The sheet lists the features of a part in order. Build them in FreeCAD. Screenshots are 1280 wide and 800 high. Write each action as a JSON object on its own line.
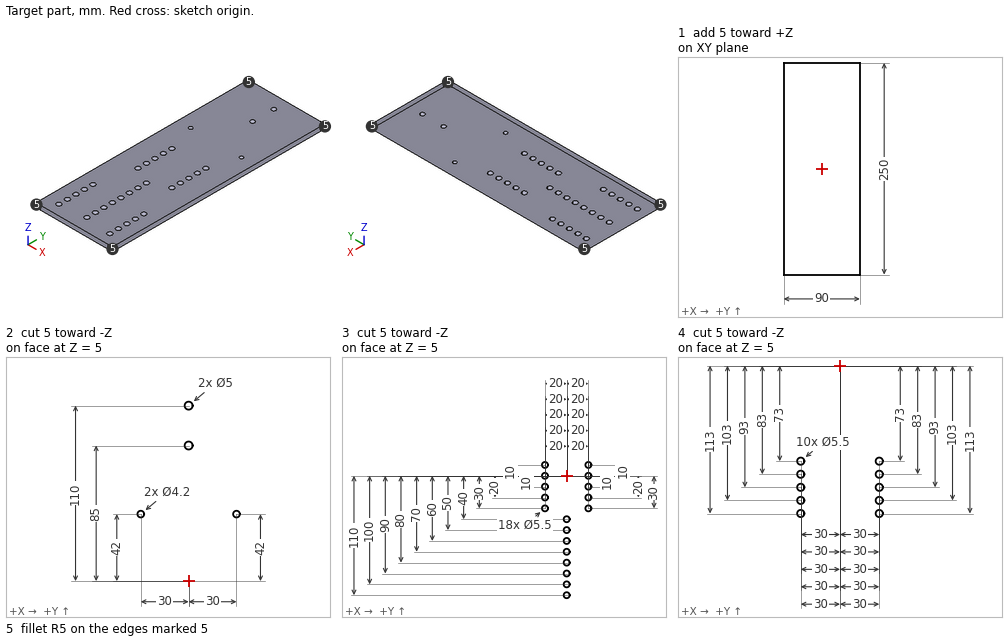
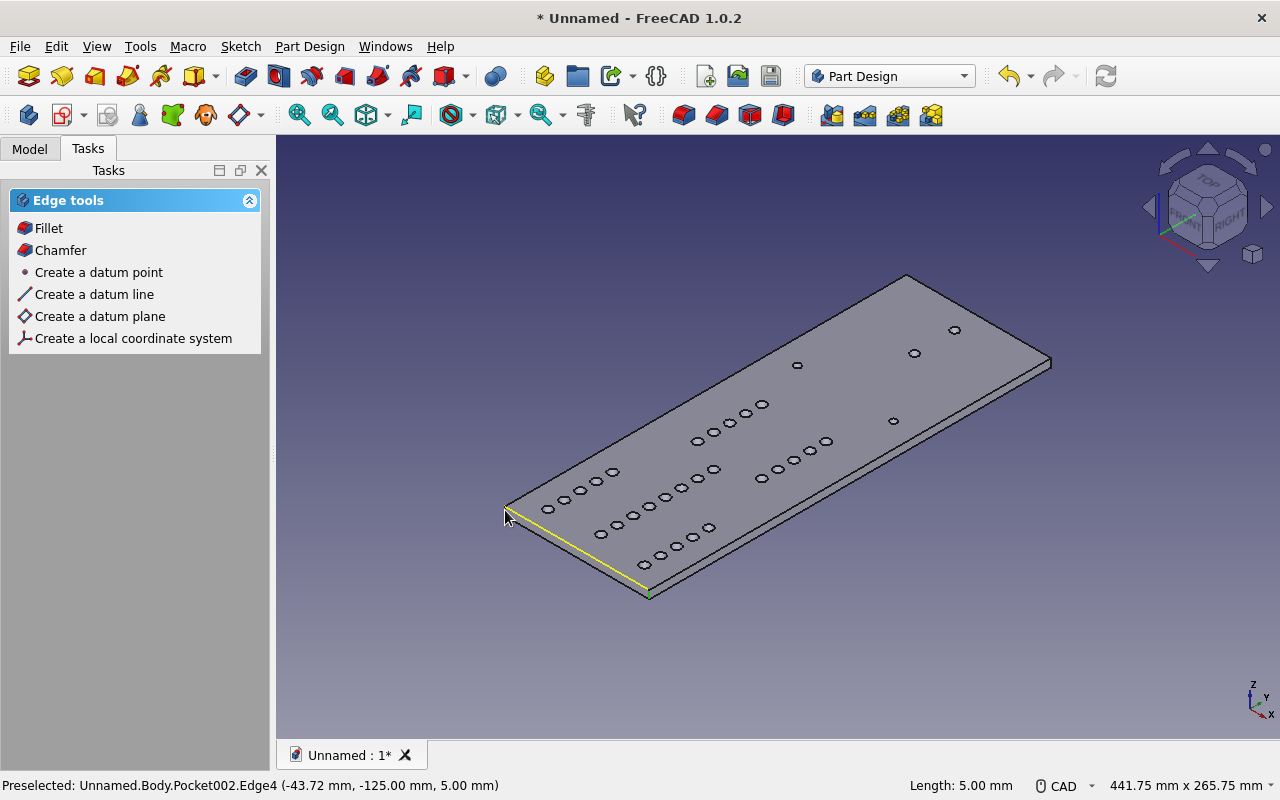
{"action": "key", "text": "2"}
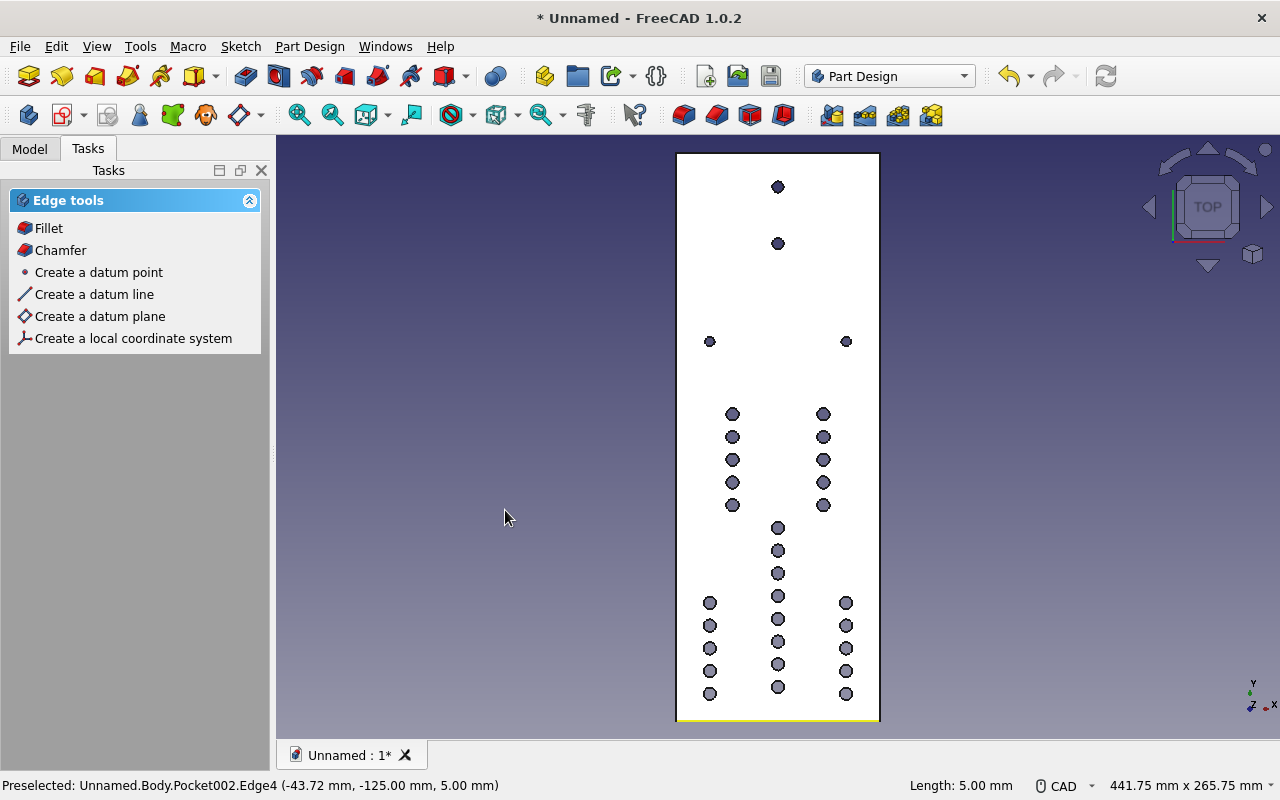
{"action": "key", "text": "1"}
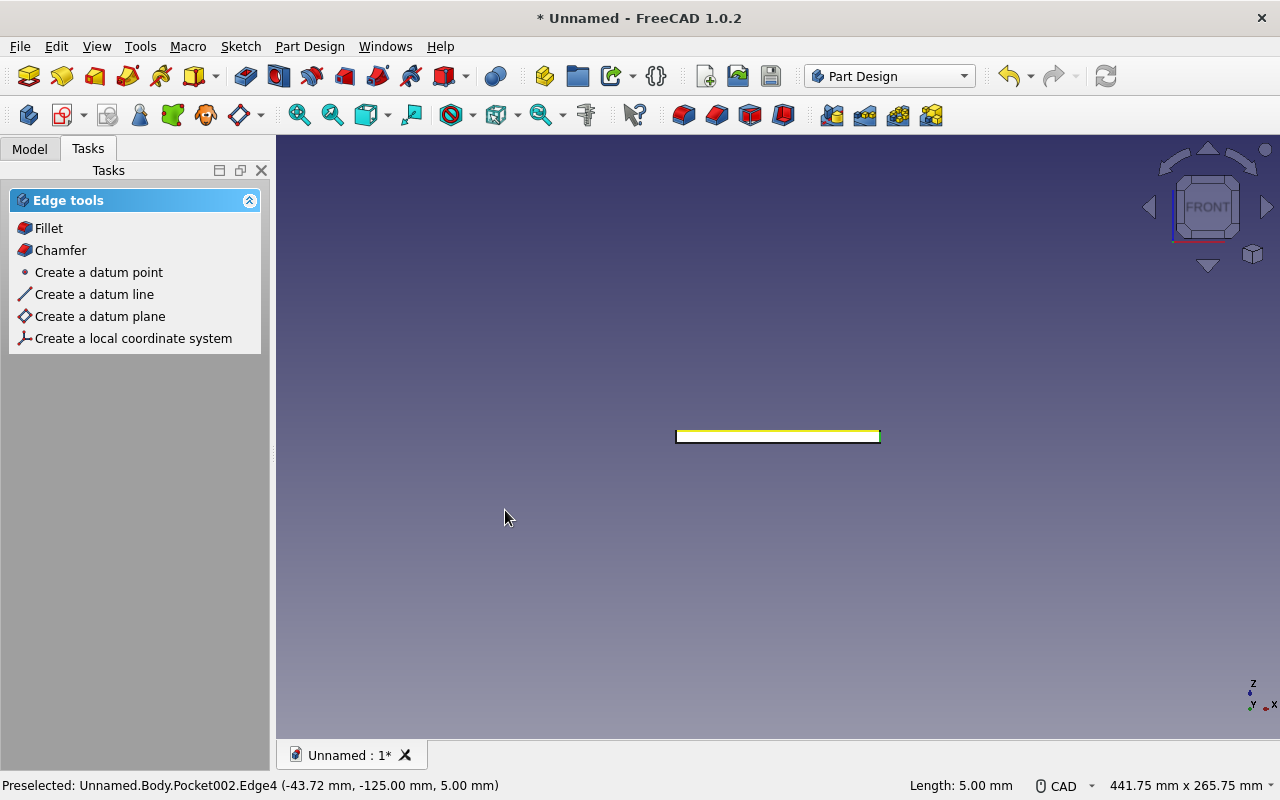
{"action": "key", "text": "v f"}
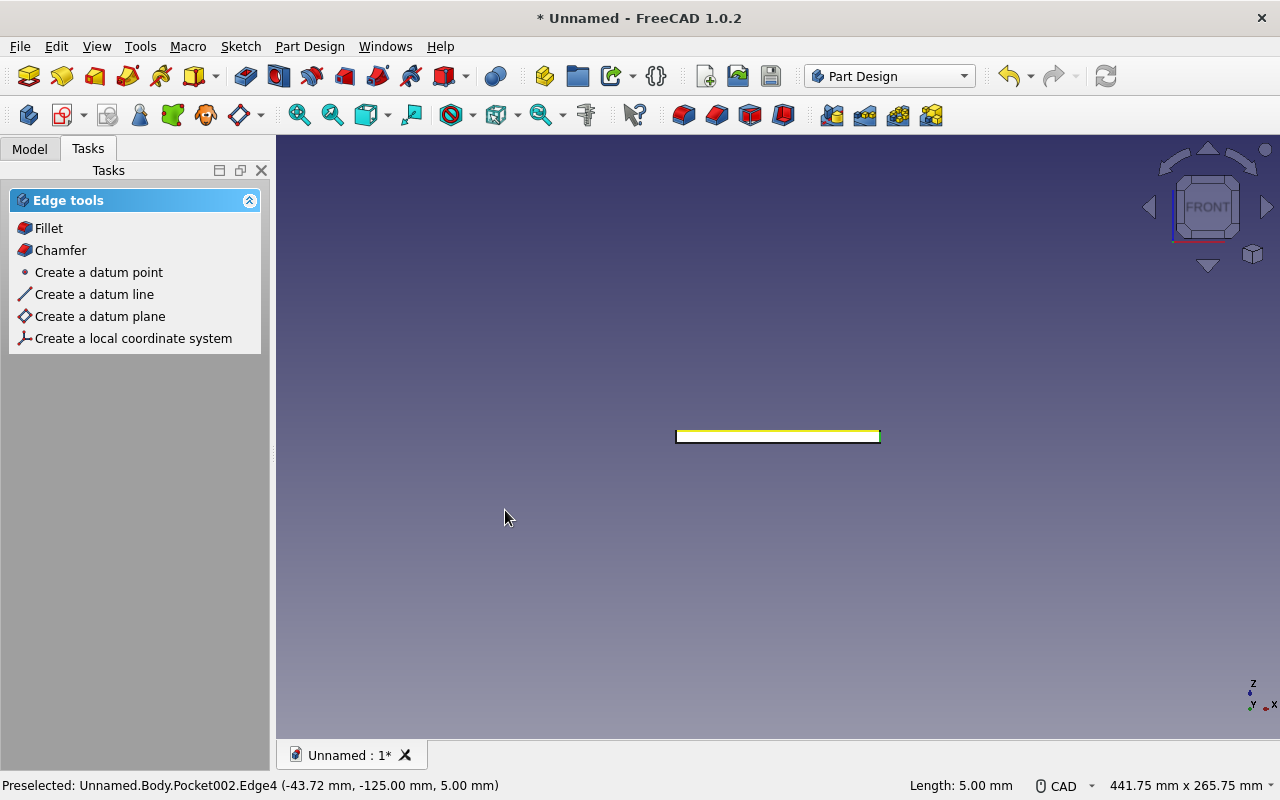
{"action": "scroll", "coordinate": [676, 436], "scroll_direction": "up", "scroll_amount": 7}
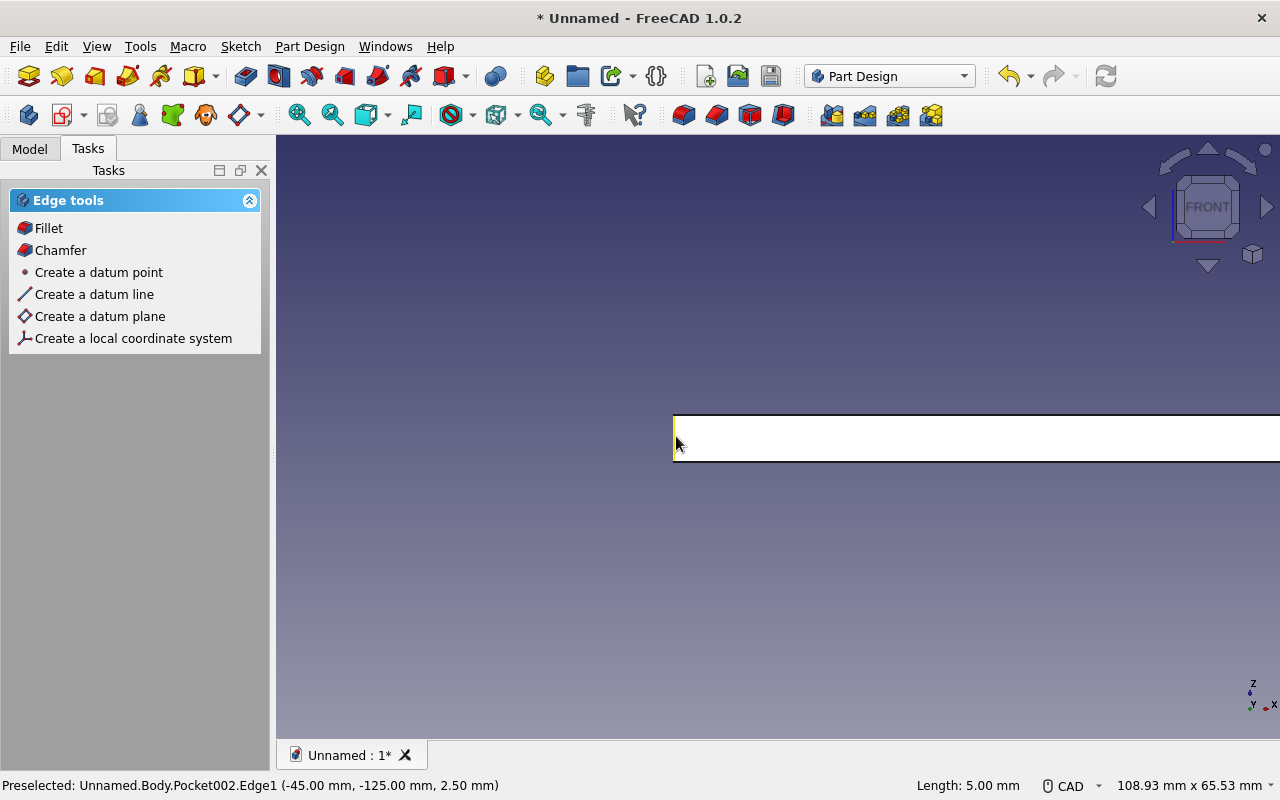
{"action": "left_click", "coordinate": [674, 438], "text": "ctrl"}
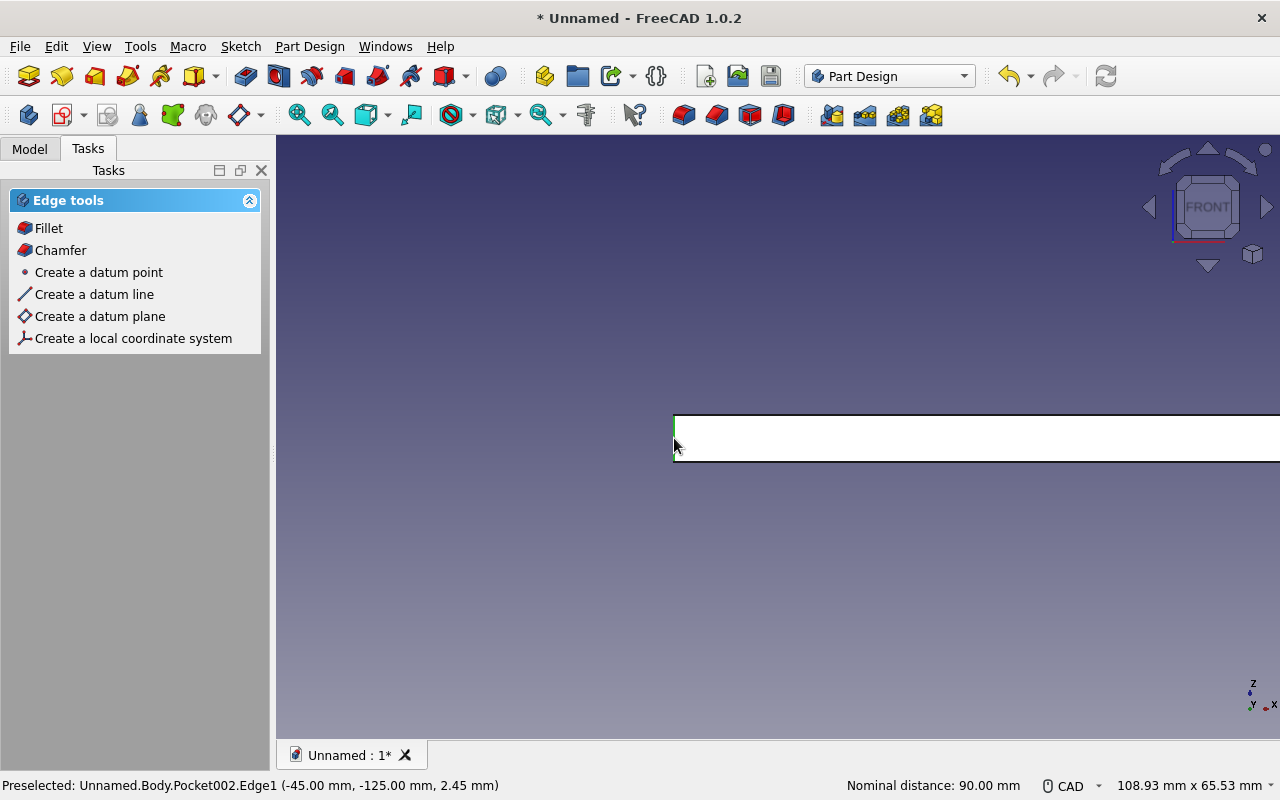
{"action": "key", "text": "v f"}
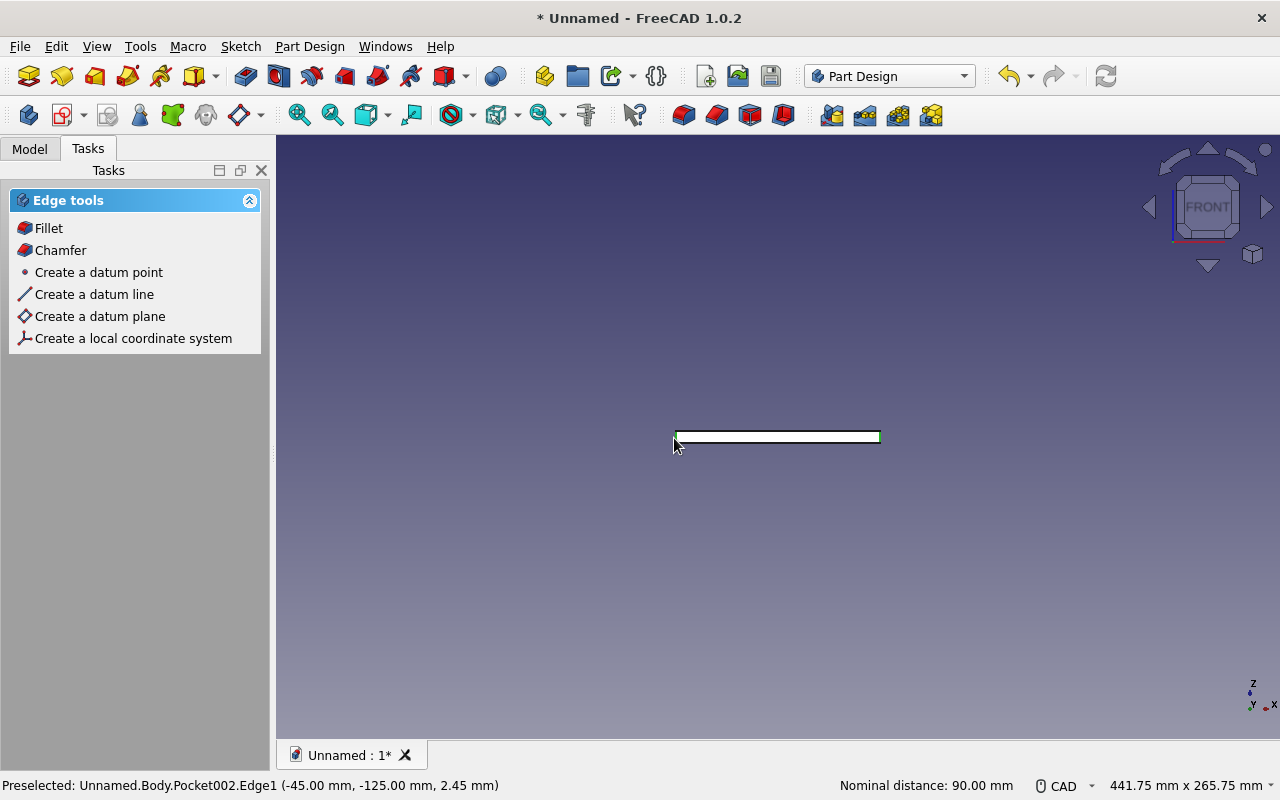
{"action": "key", "text": "3"}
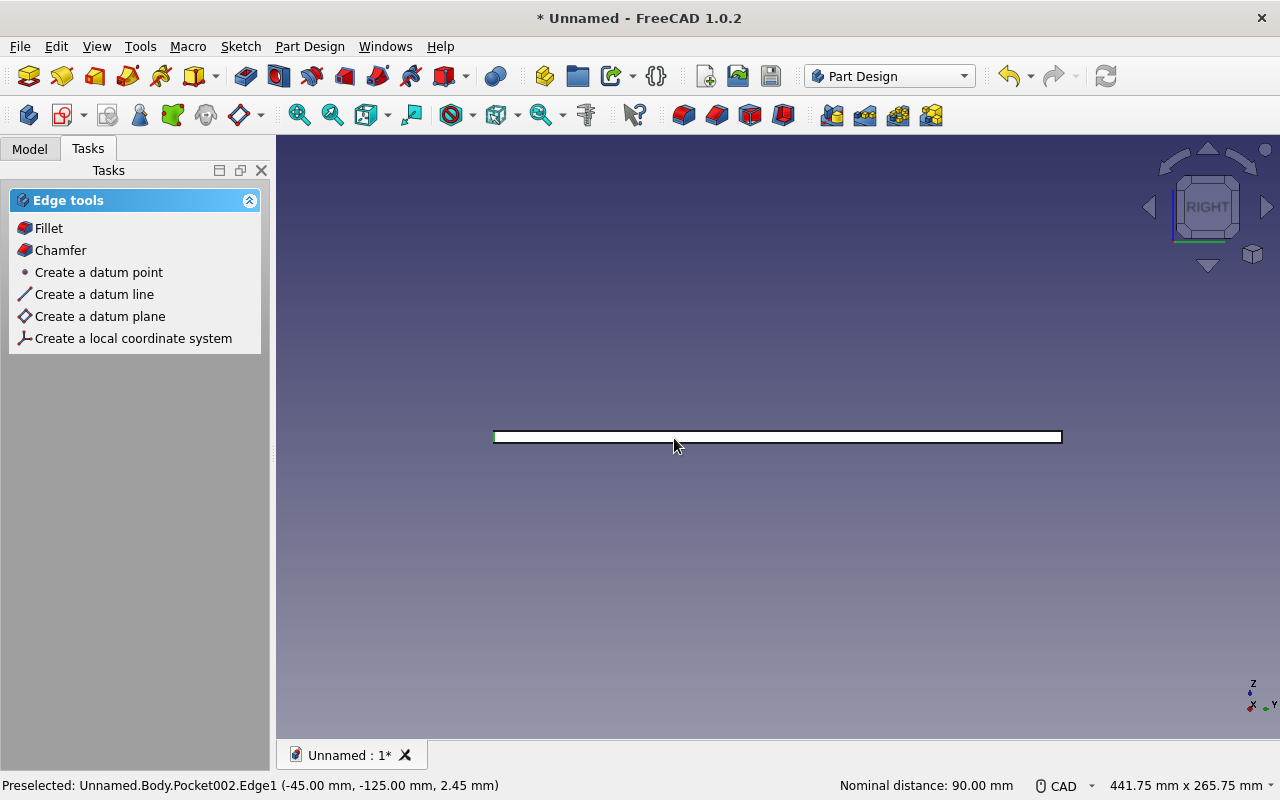
{"action": "scroll", "coordinate": [1062, 436], "scroll_direction": "up", "scroll_amount": 7}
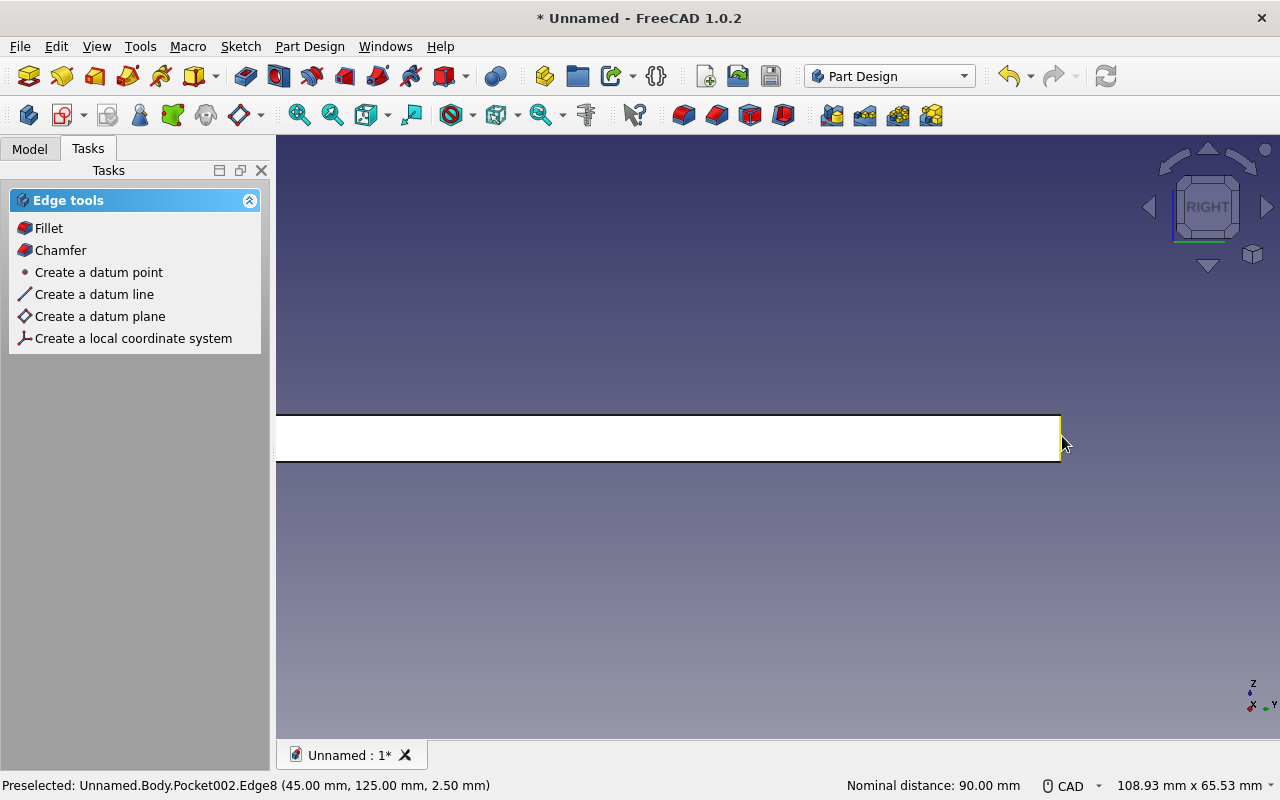
{"action": "left_click", "coordinate": [1060, 438], "text": "ctrl"}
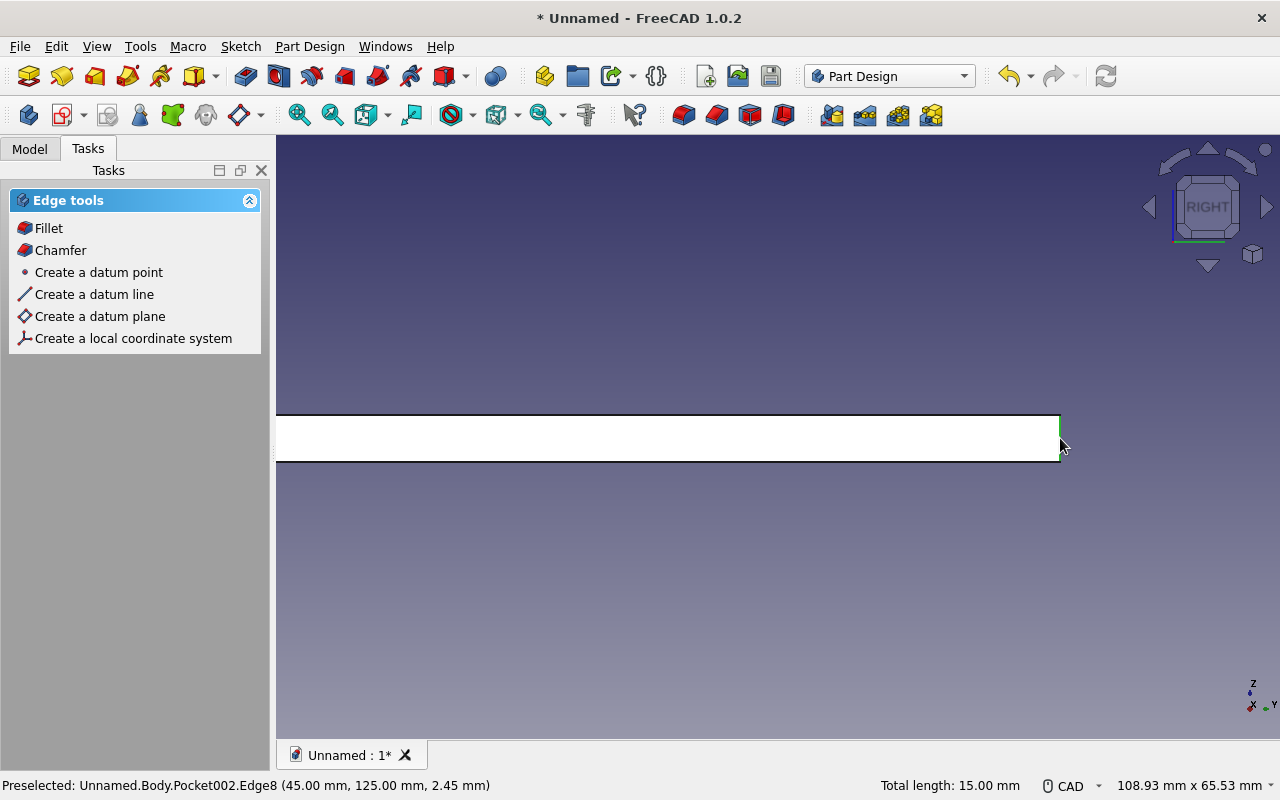
{"action": "left_click", "coordinate": [300, 116]}